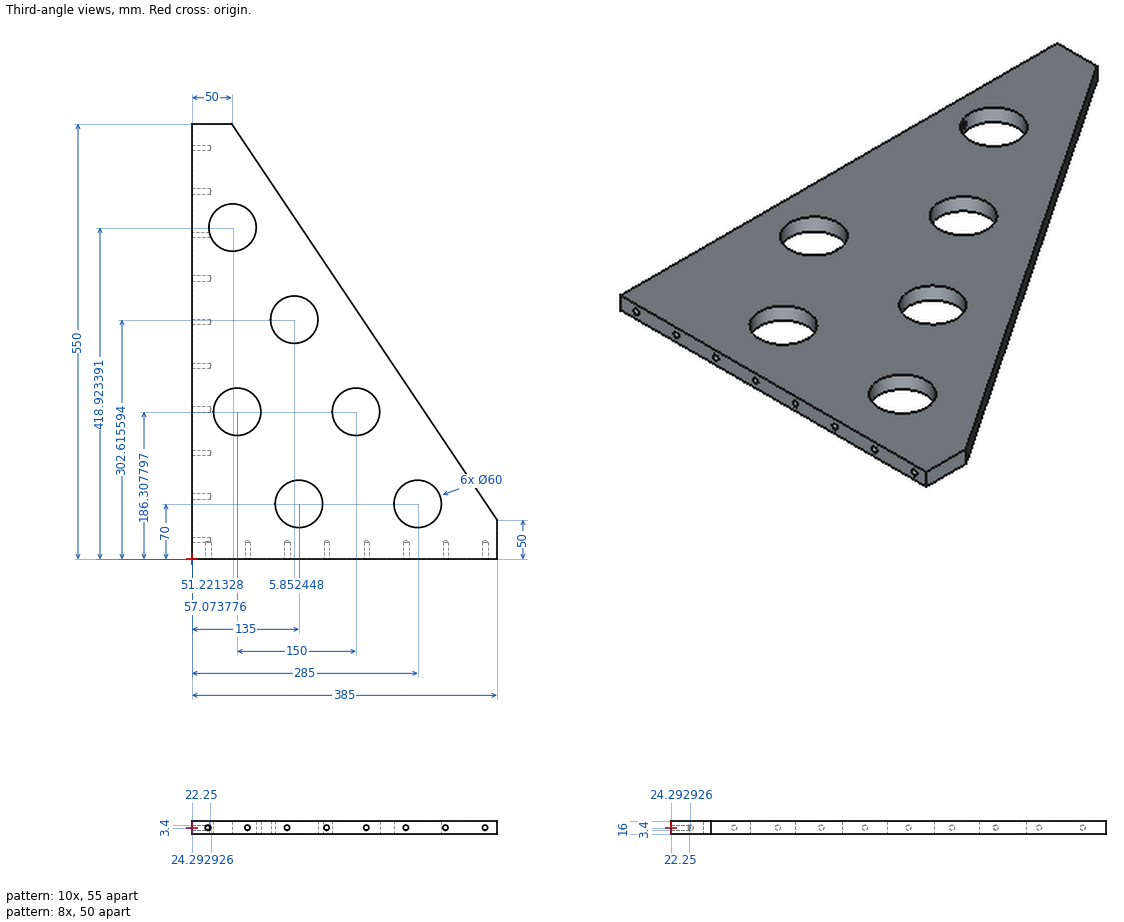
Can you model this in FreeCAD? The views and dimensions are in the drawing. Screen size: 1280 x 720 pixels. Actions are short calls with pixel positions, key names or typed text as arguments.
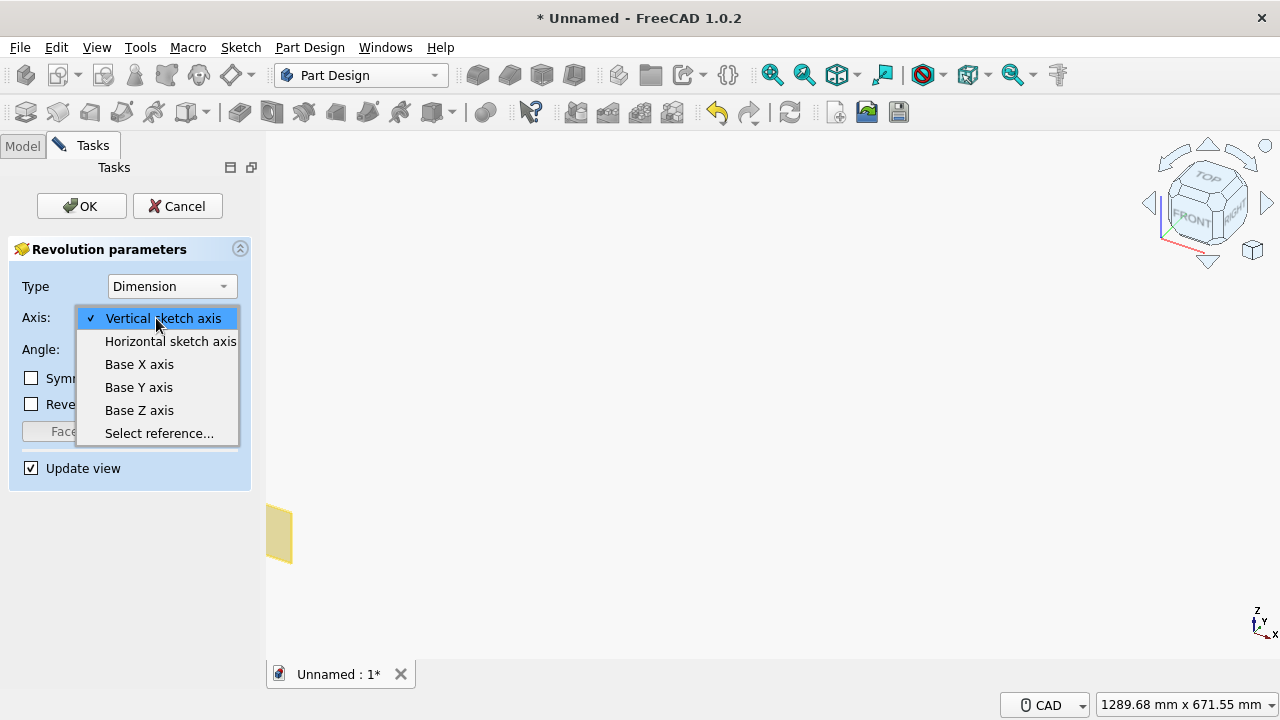
click(156, 342)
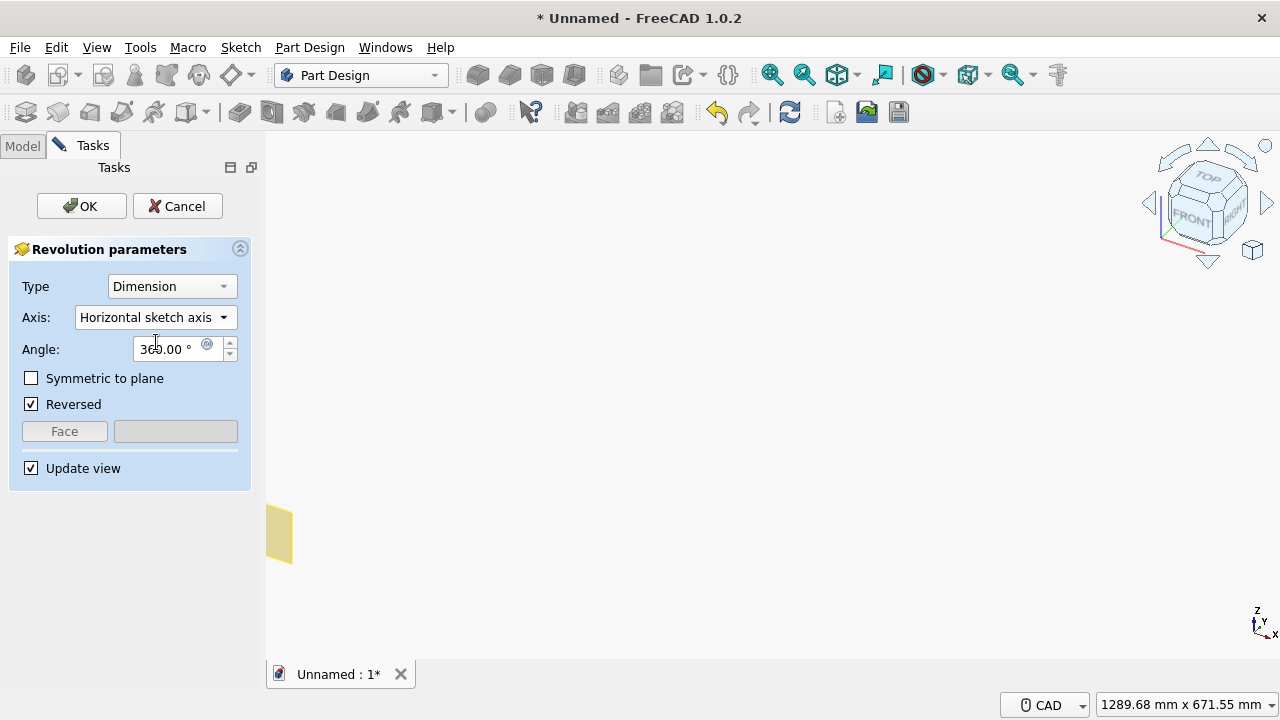
click(82, 206)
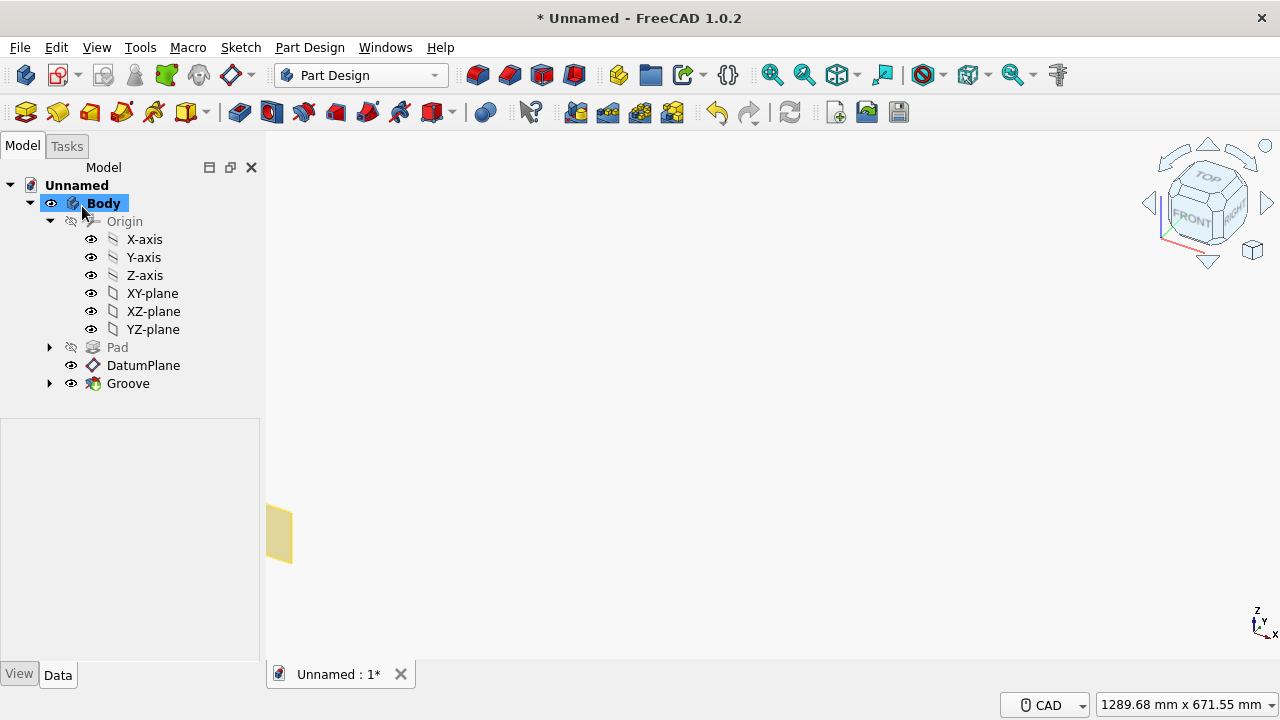
click(116, 365)
key(space)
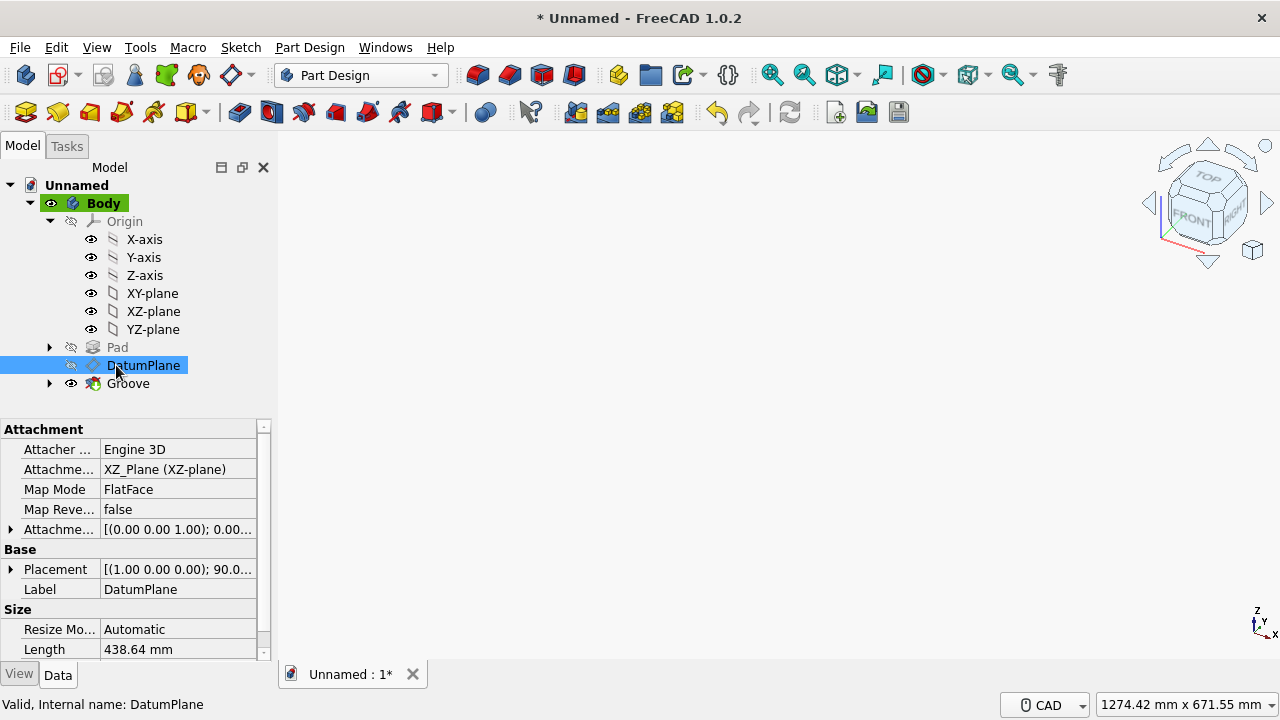
click(774, 76)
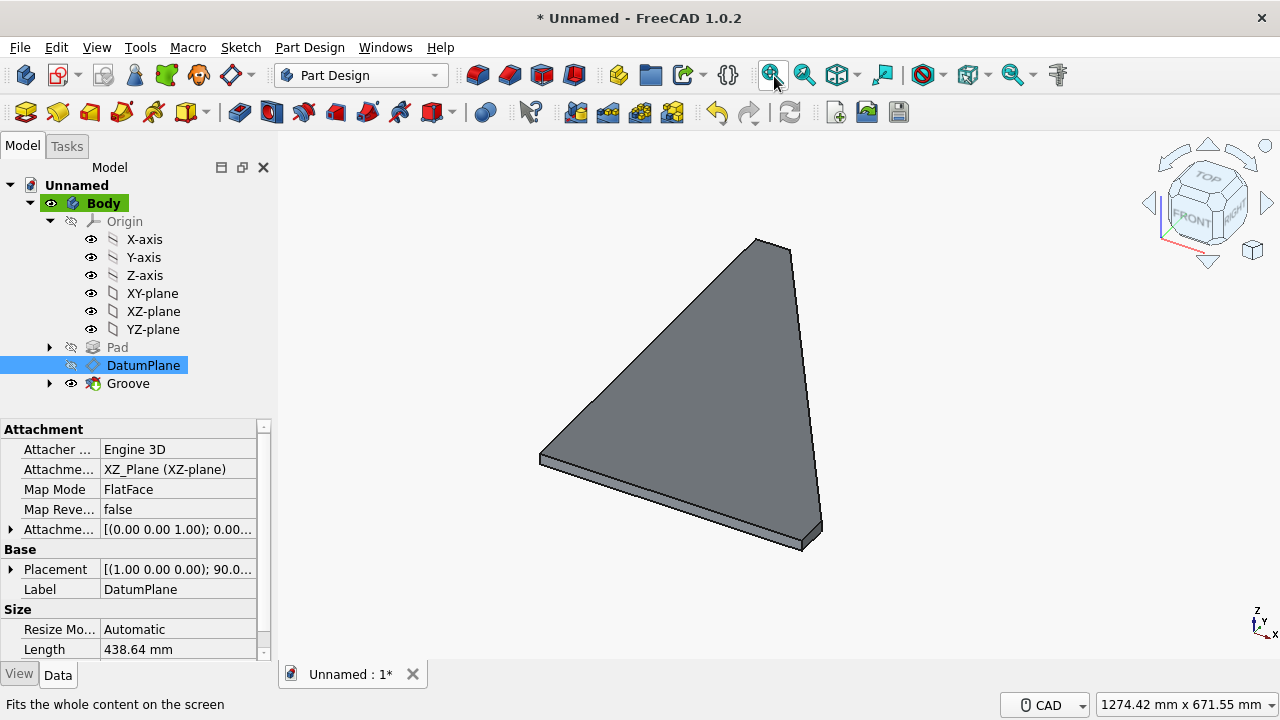
click(116, 383)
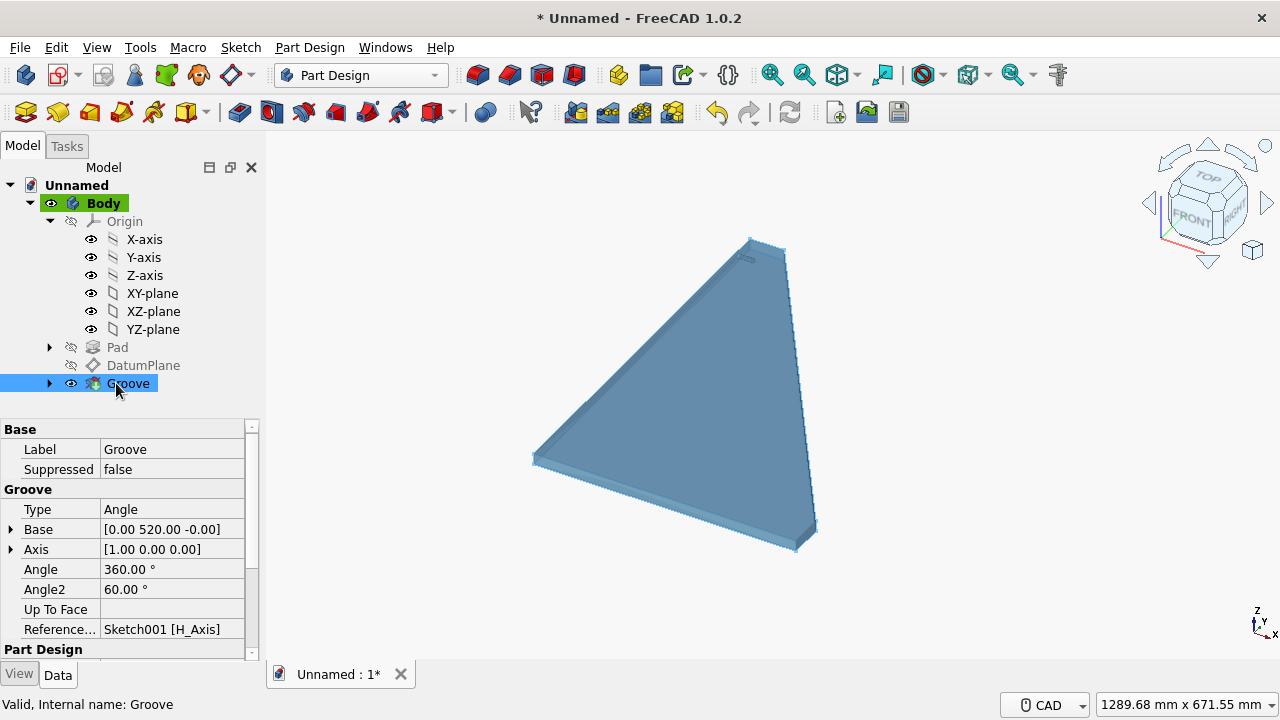
click(608, 112)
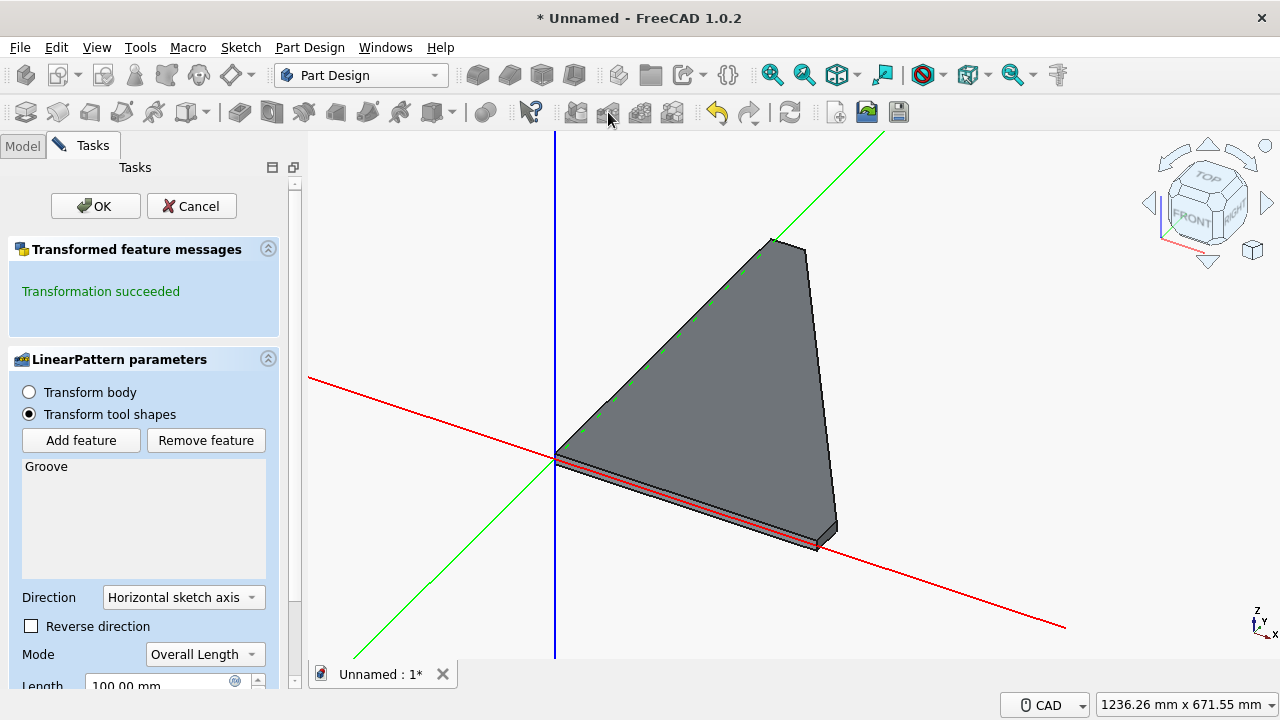
click(184, 598)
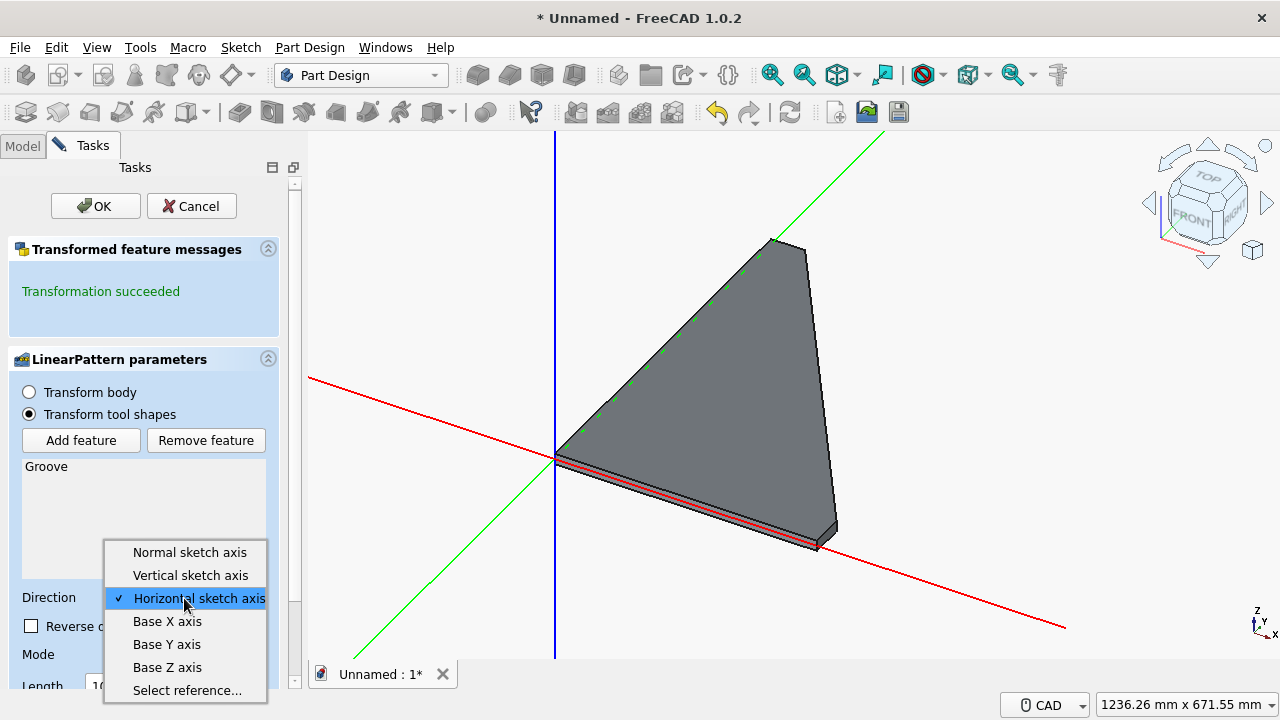
click(184, 644)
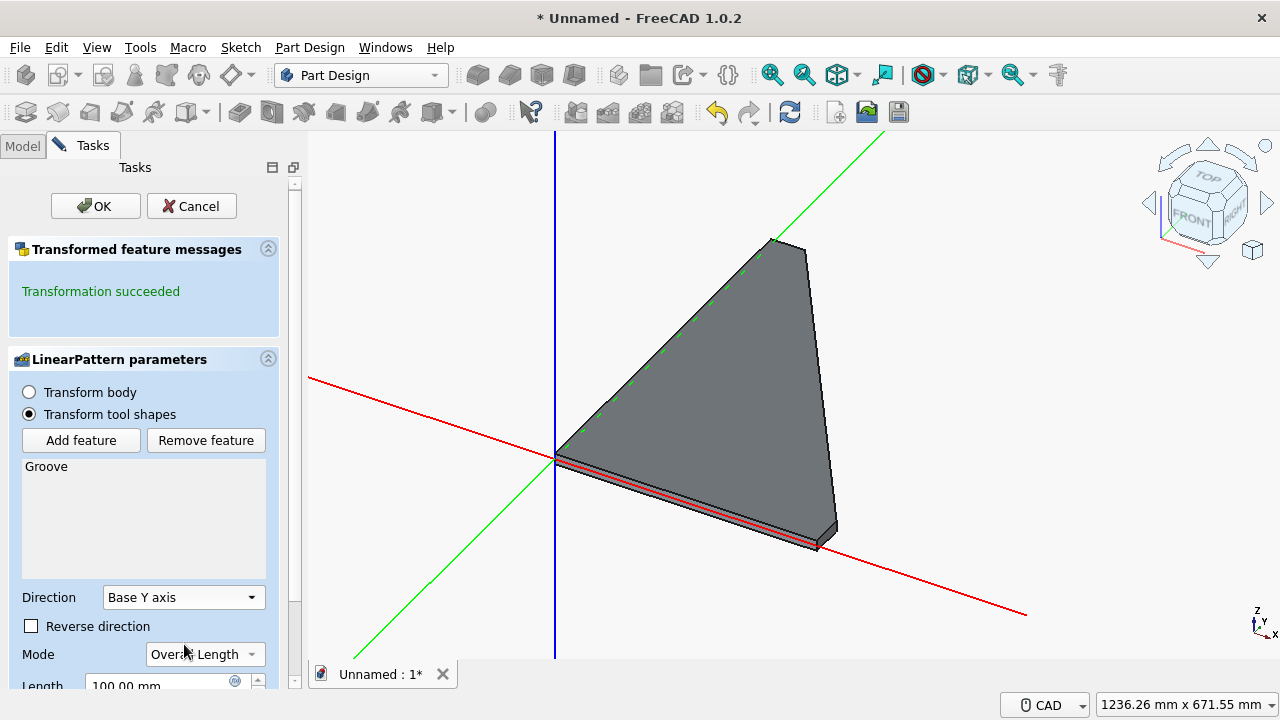
click(206, 654)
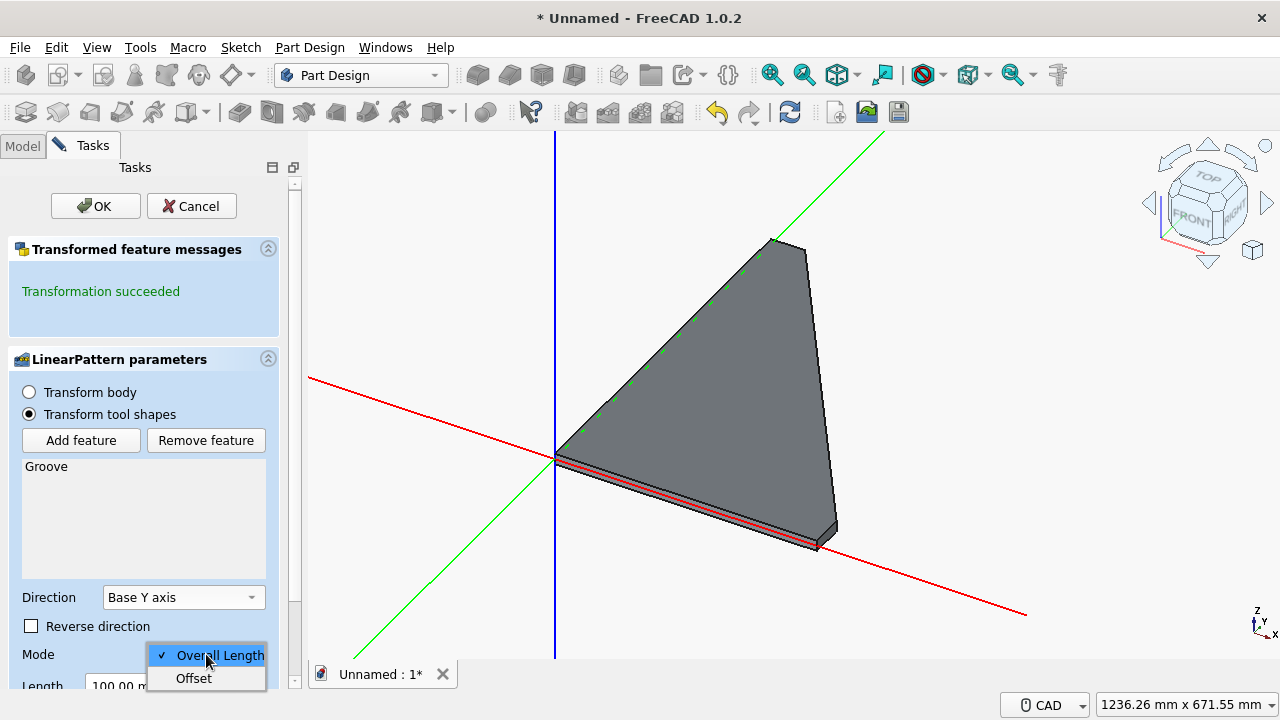
click(206, 678)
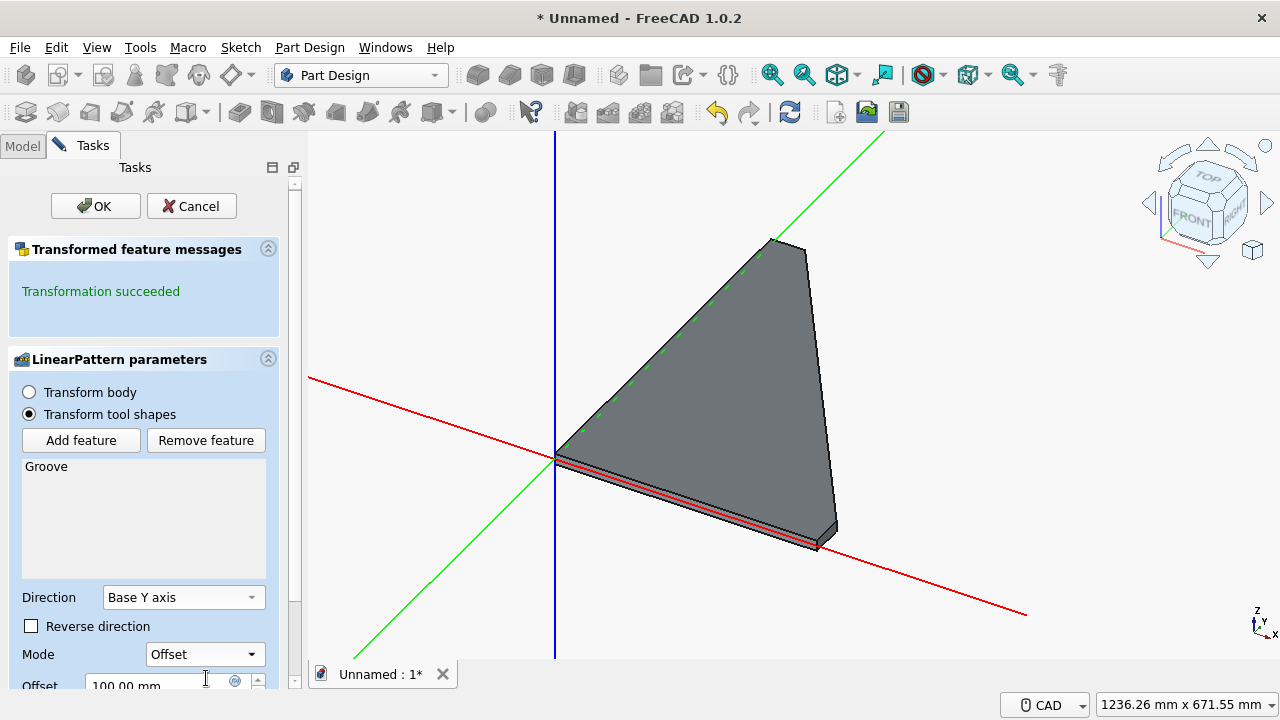
scroll(295, 432, down, 2)